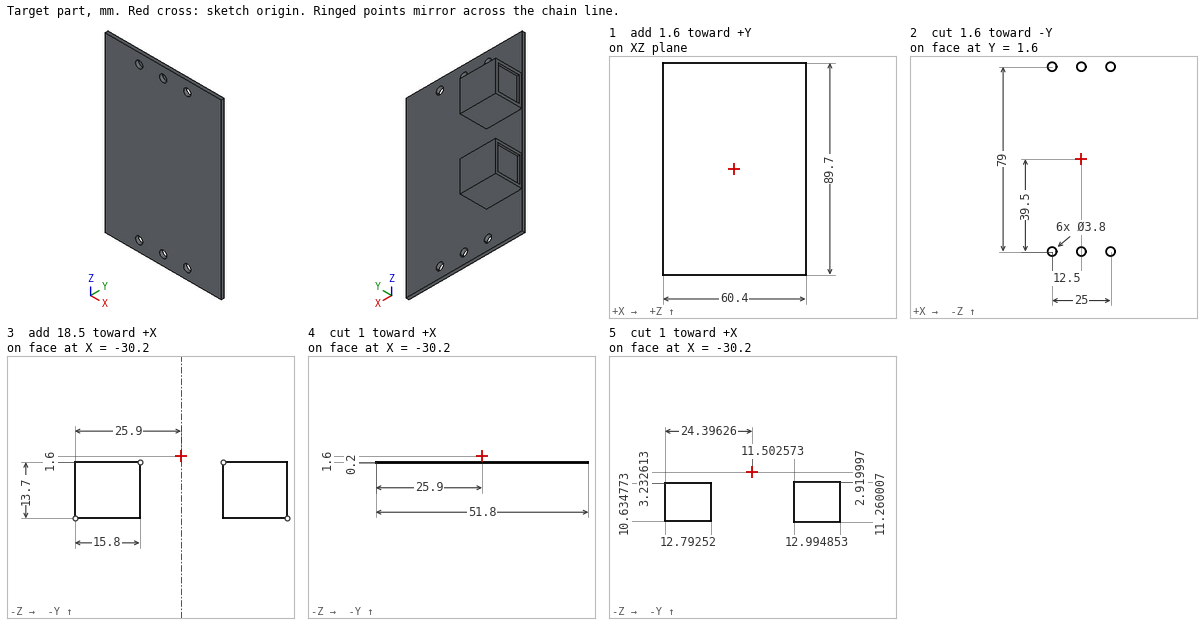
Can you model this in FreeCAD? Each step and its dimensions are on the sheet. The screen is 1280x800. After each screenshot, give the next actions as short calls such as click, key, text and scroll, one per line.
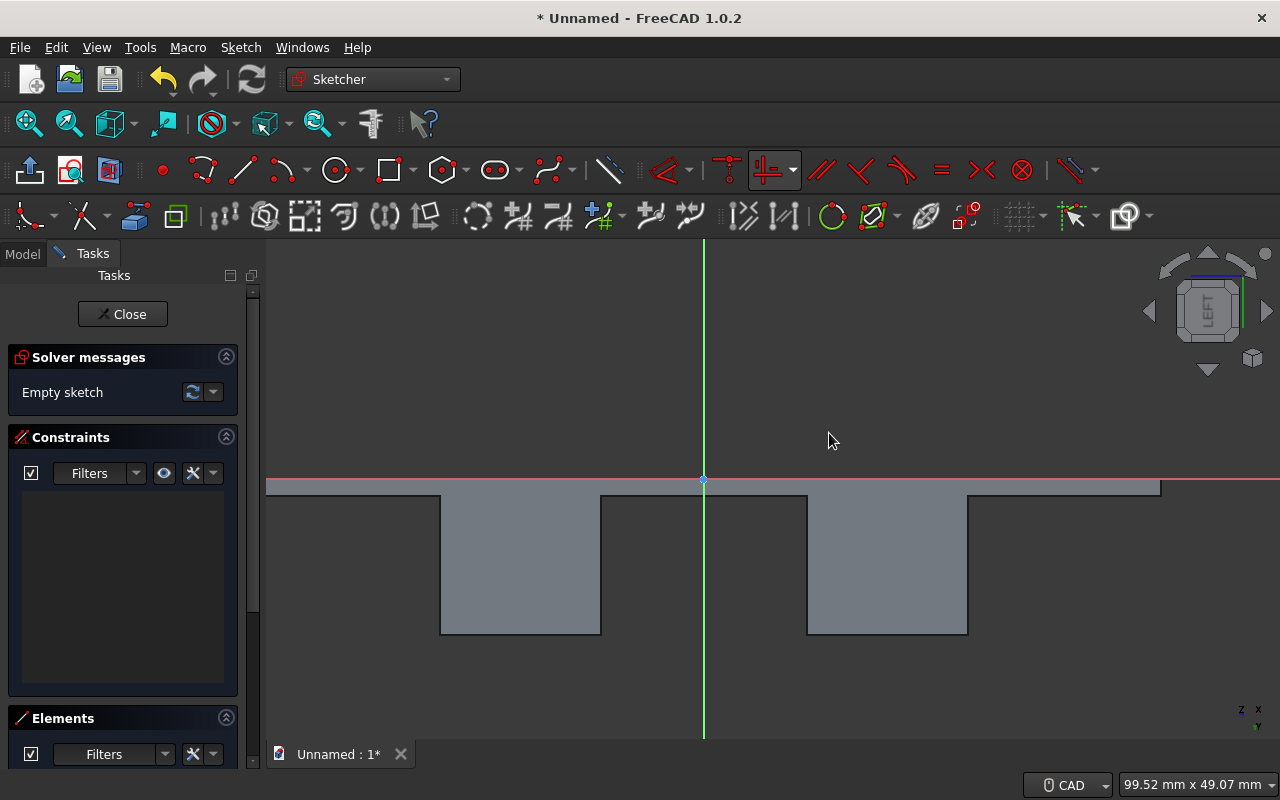
key(g)
key(r)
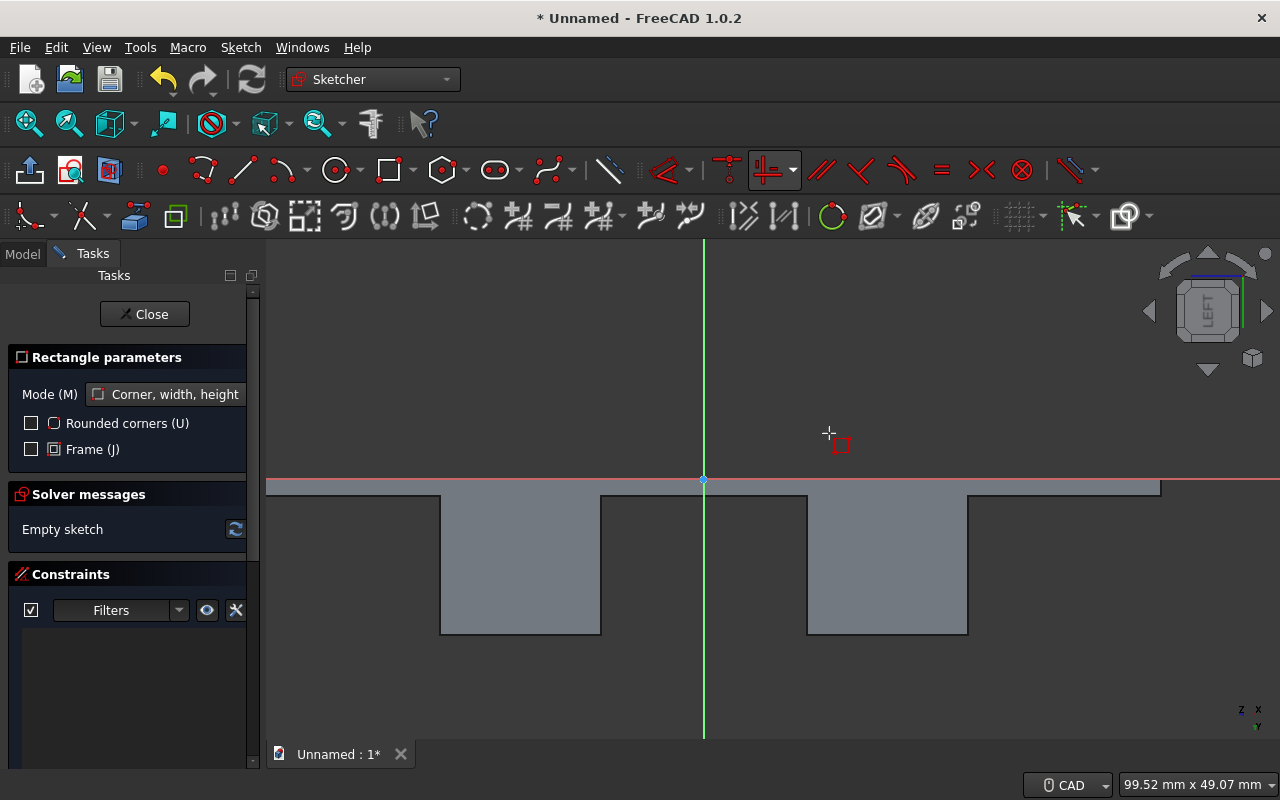
scroll(440, 496, up, 11)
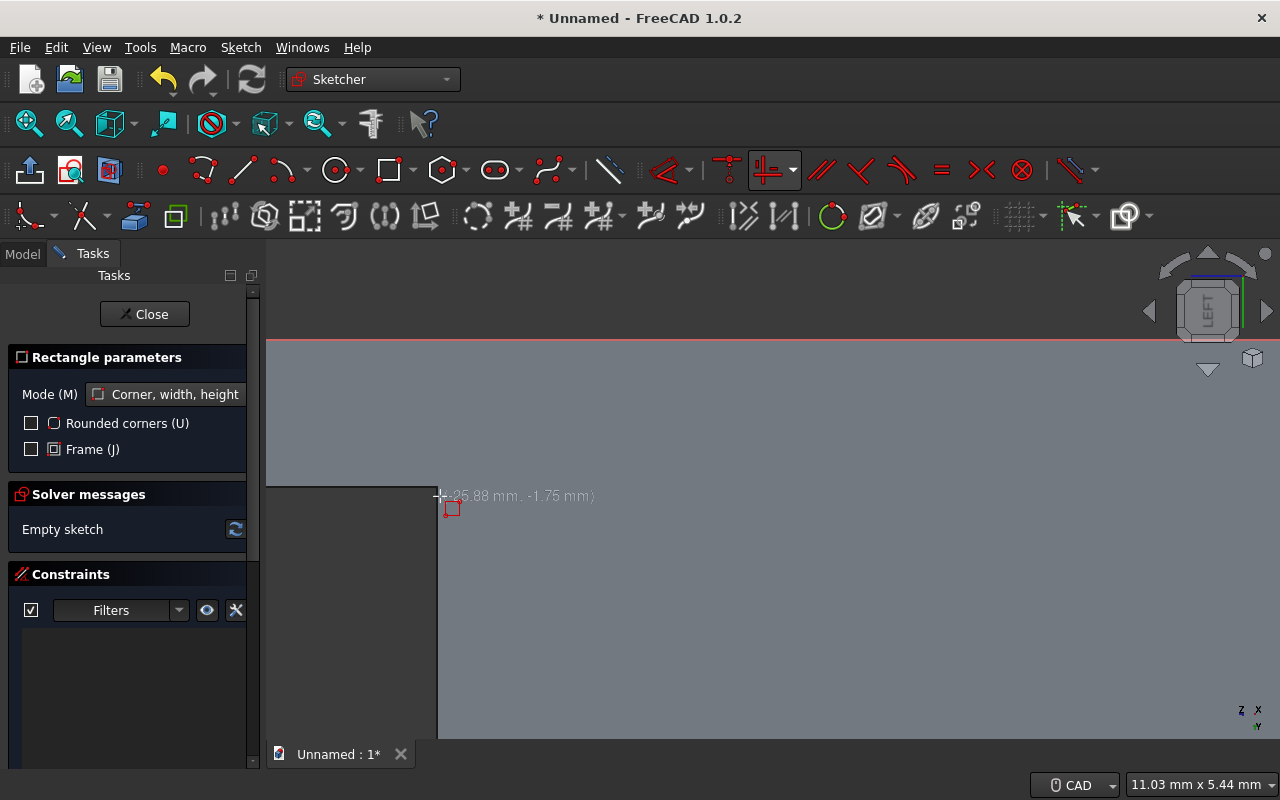
scroll(441, 497, down, 11)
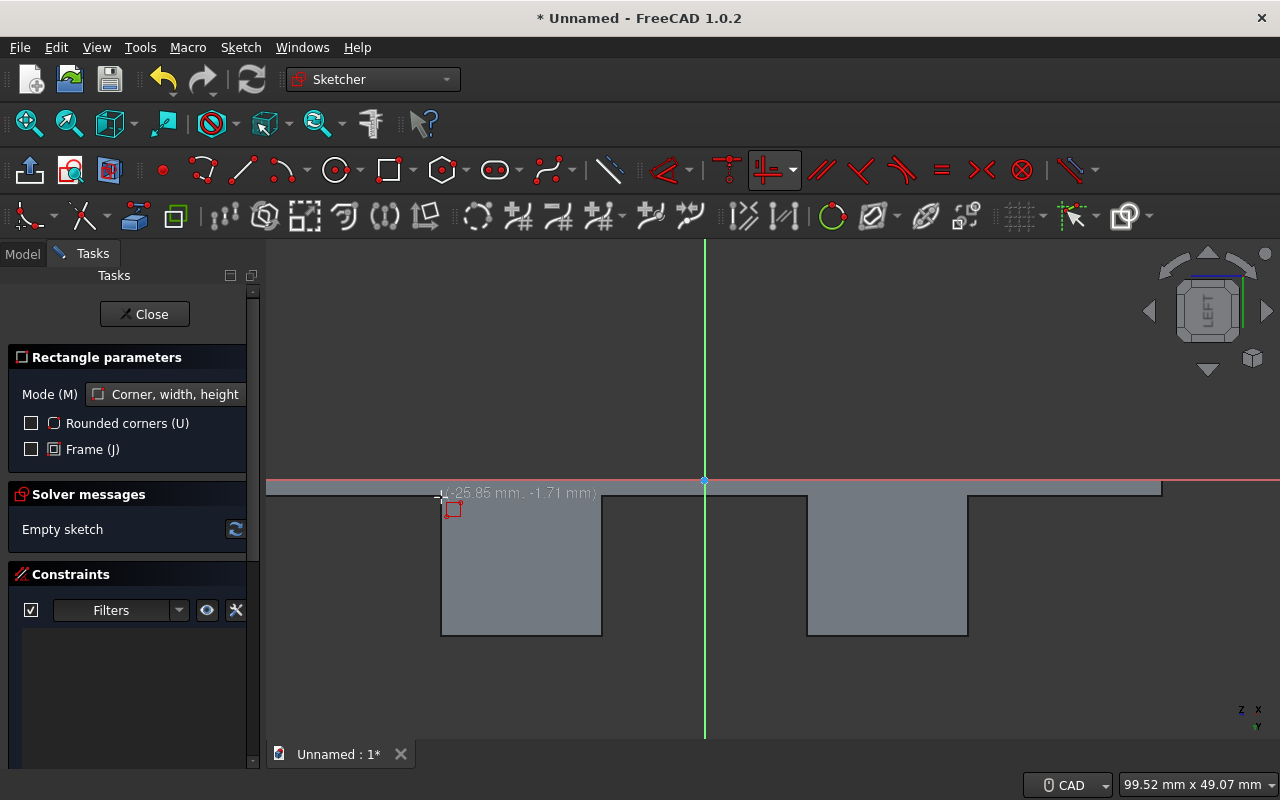
click(441, 496)
click(968, 498)
key(Escape)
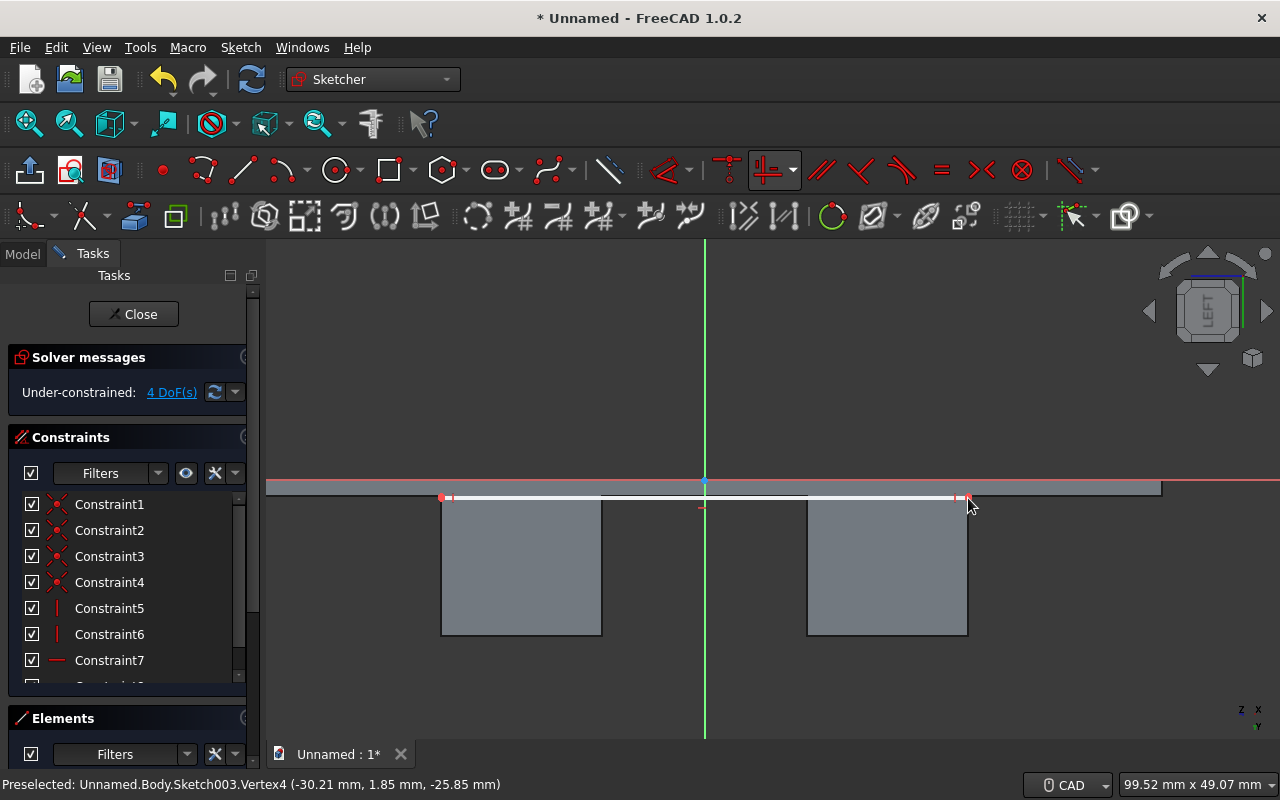
key(d)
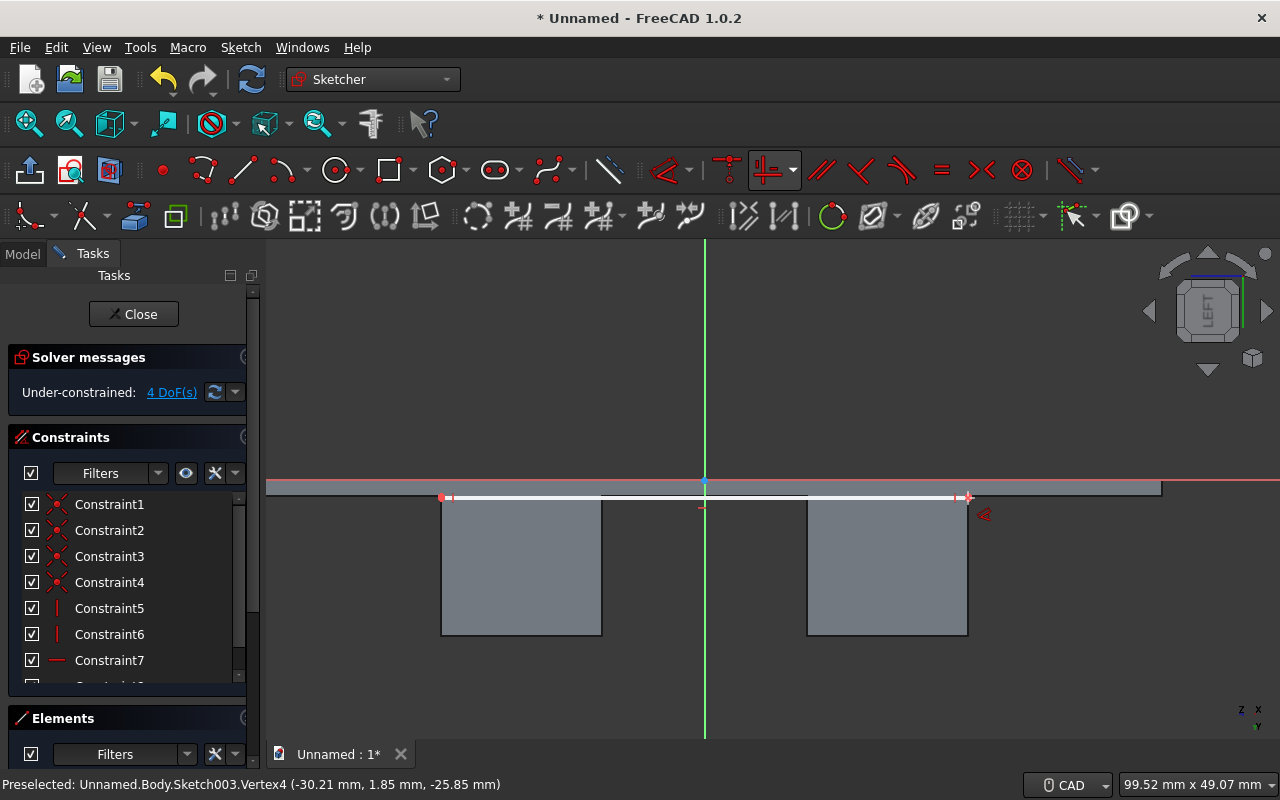
scroll(441, 498, up, 15)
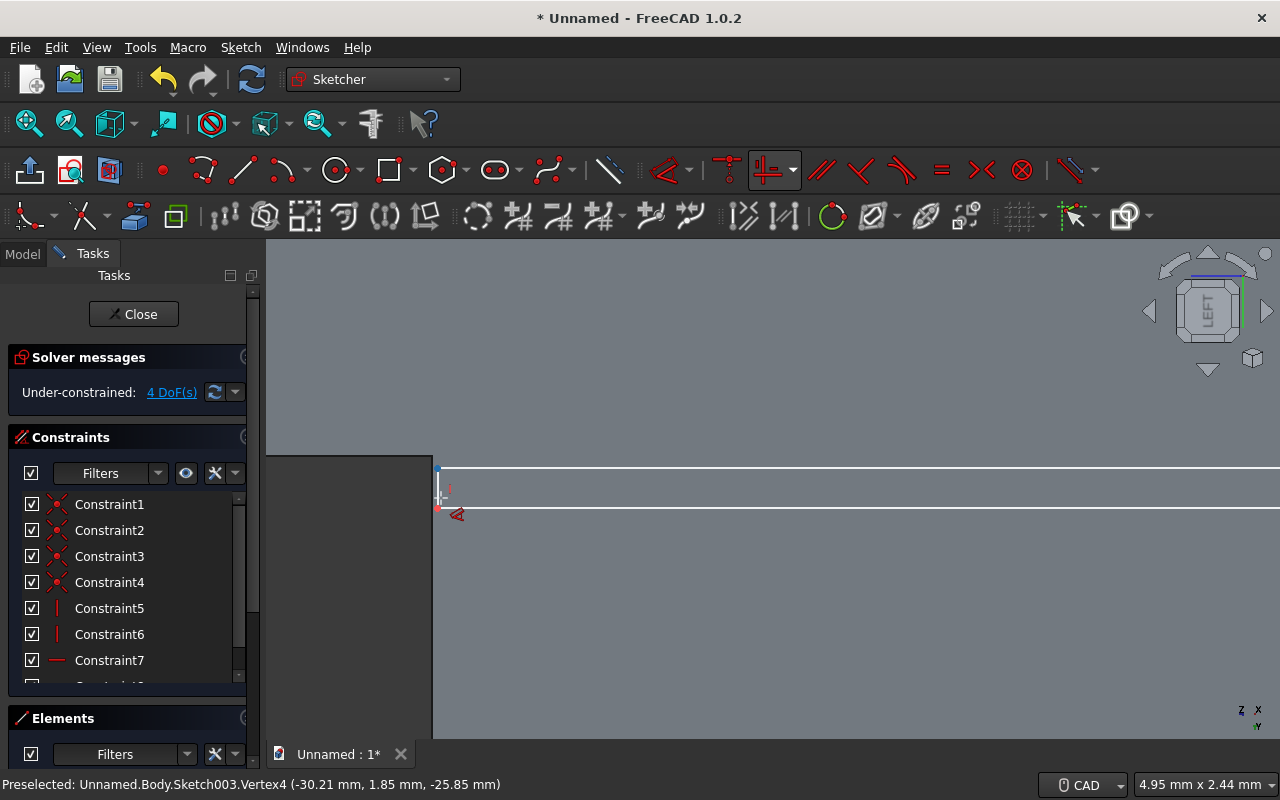
click(438, 488)
click(404, 488)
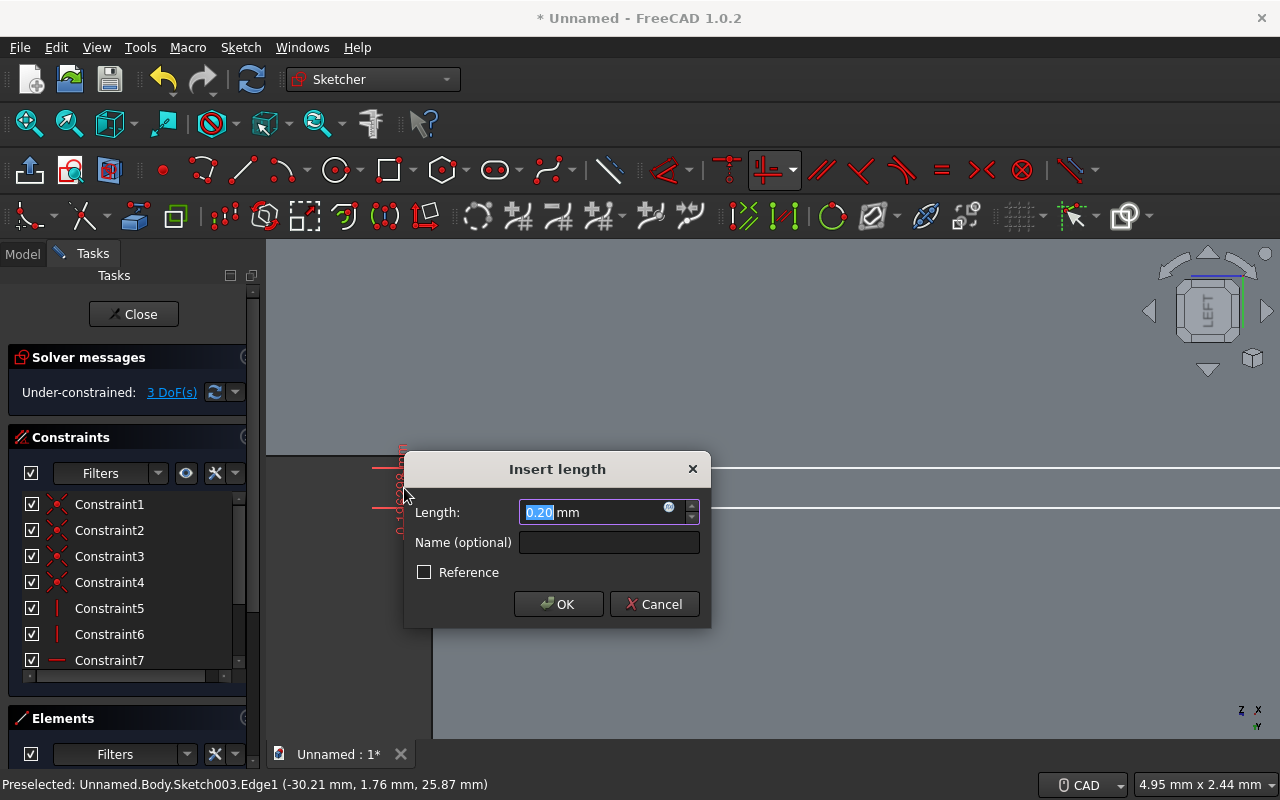
text(0.2)
key(Return)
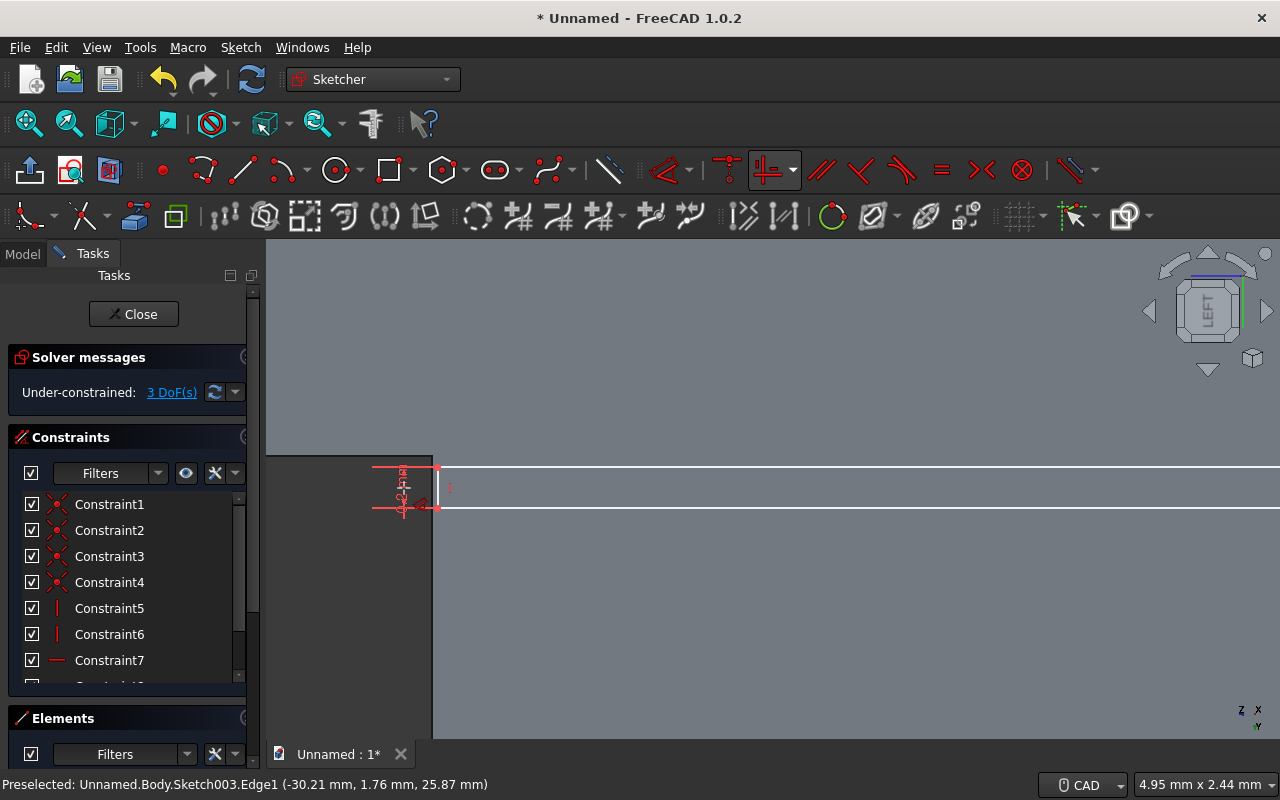
scroll(441, 498, down, 15)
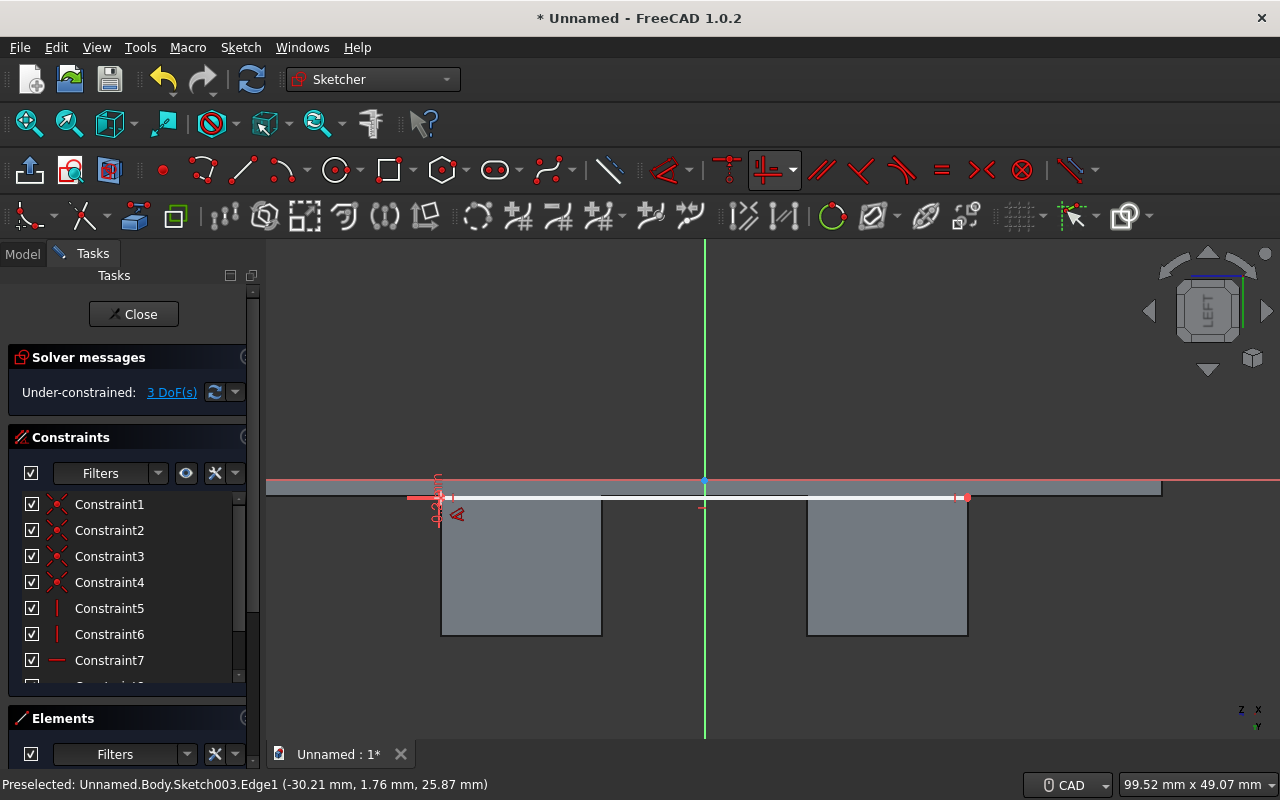
scroll(599, 499, up, 10)